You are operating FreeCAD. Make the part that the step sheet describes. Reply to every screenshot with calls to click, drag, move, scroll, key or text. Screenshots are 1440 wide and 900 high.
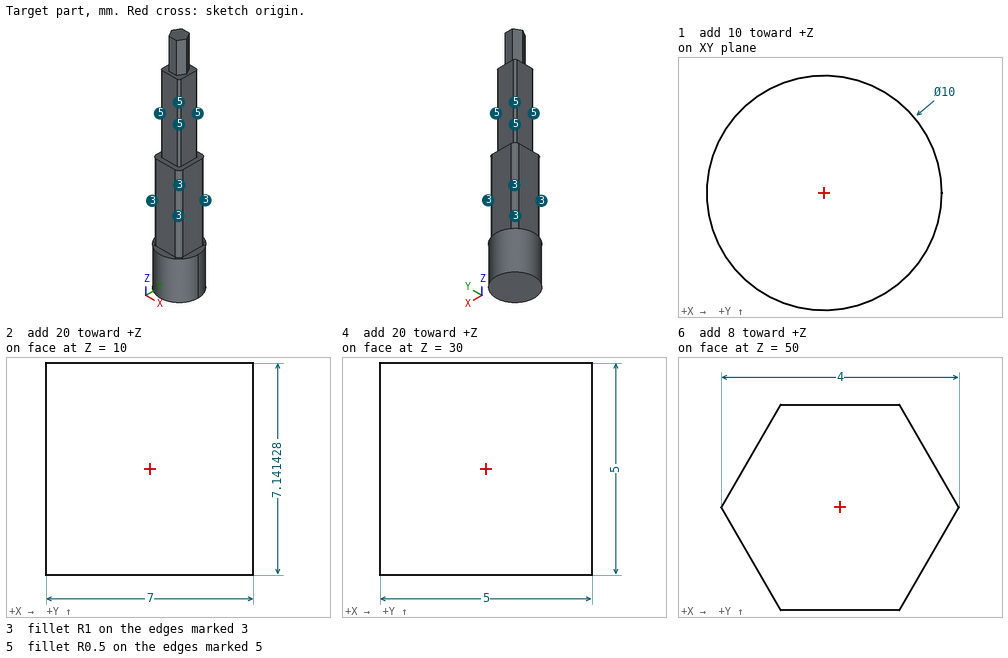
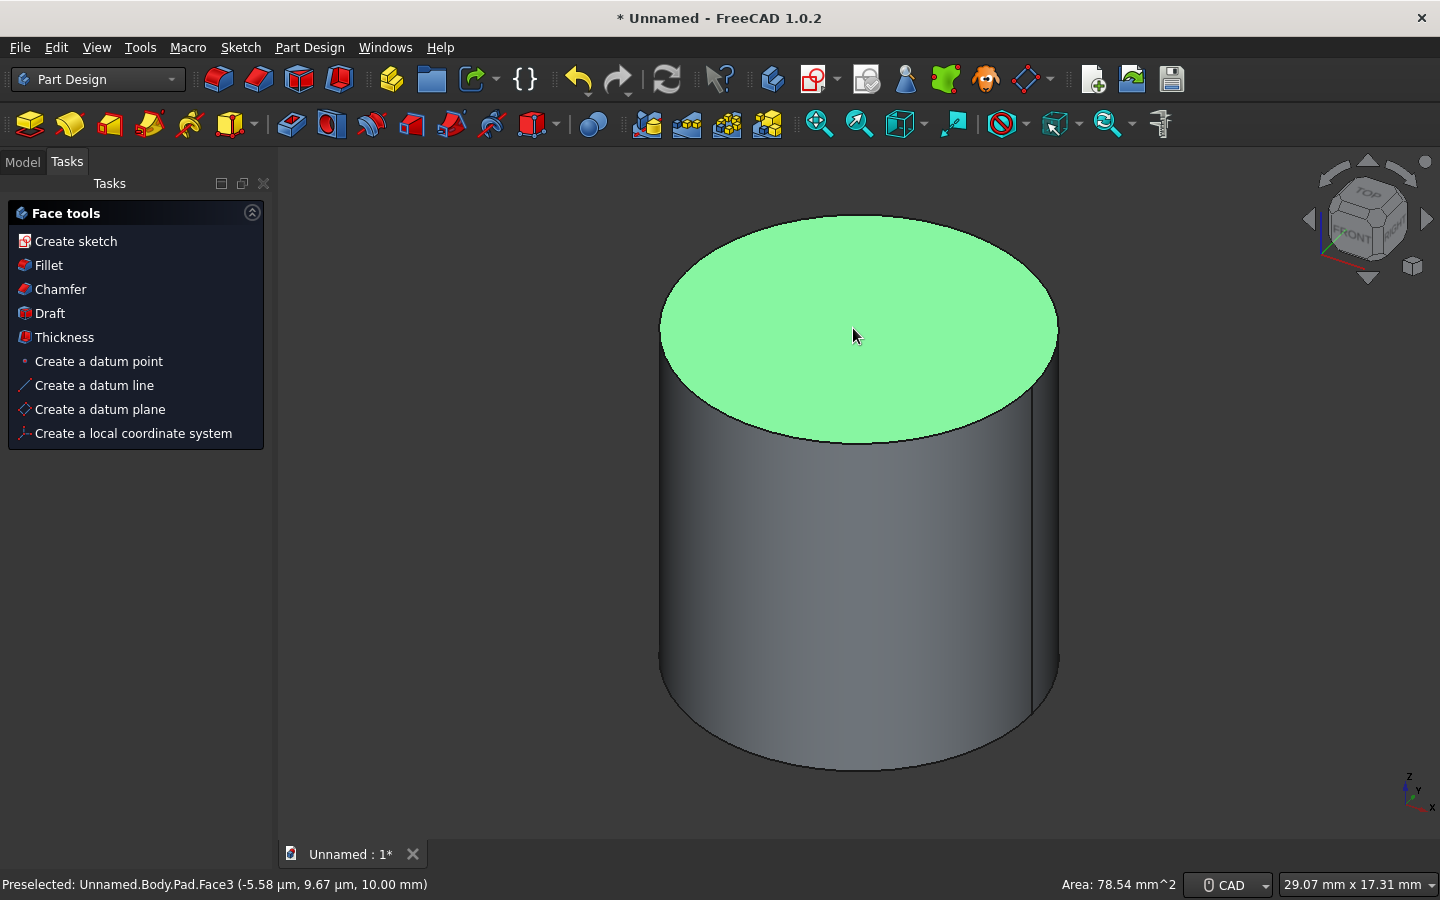
click(814, 80)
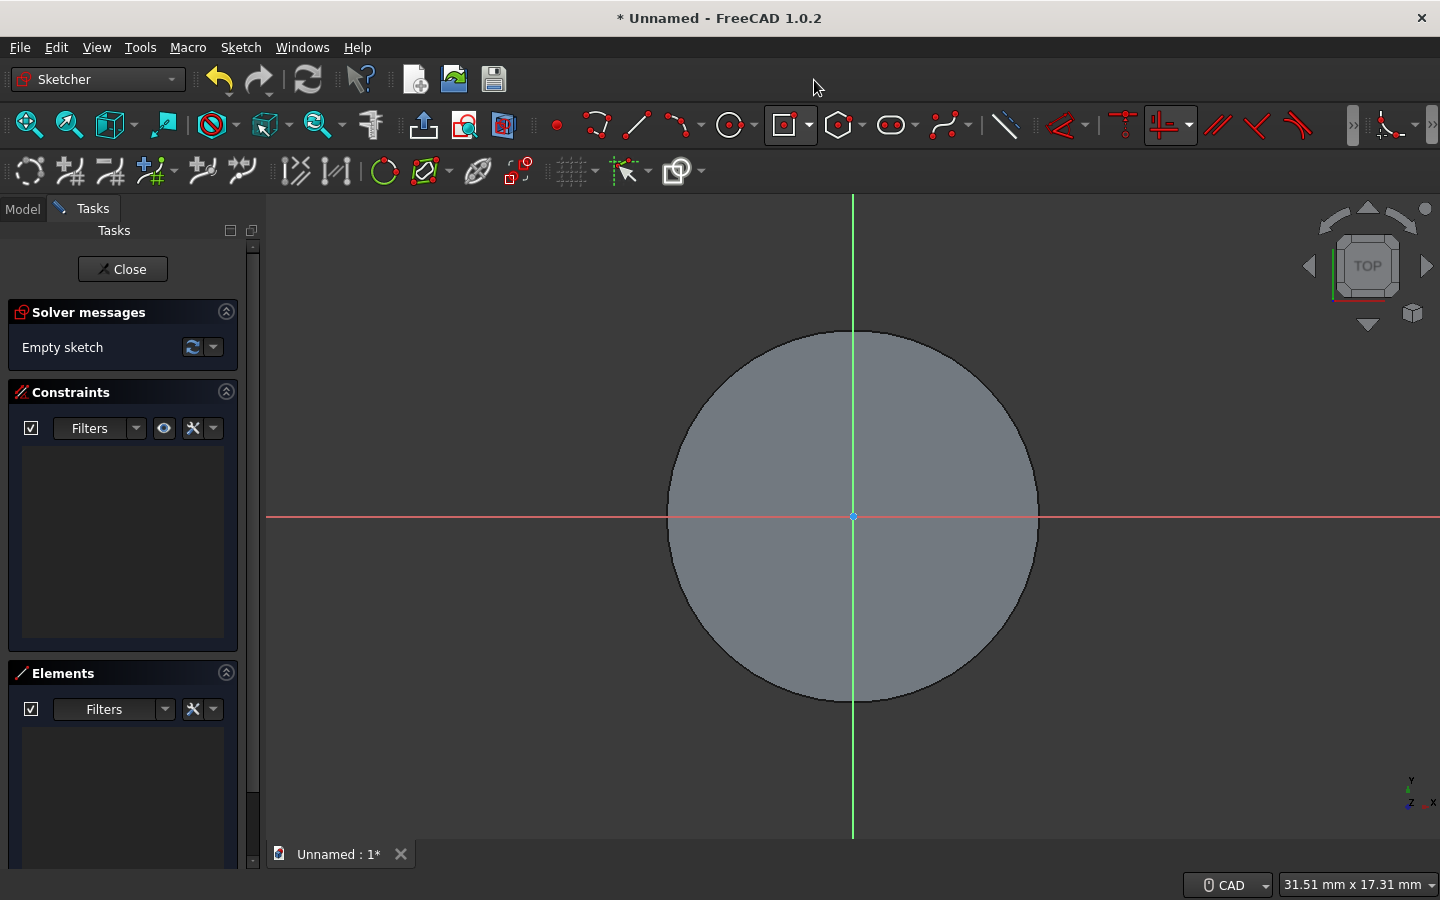
scroll(992, 517, up, 2)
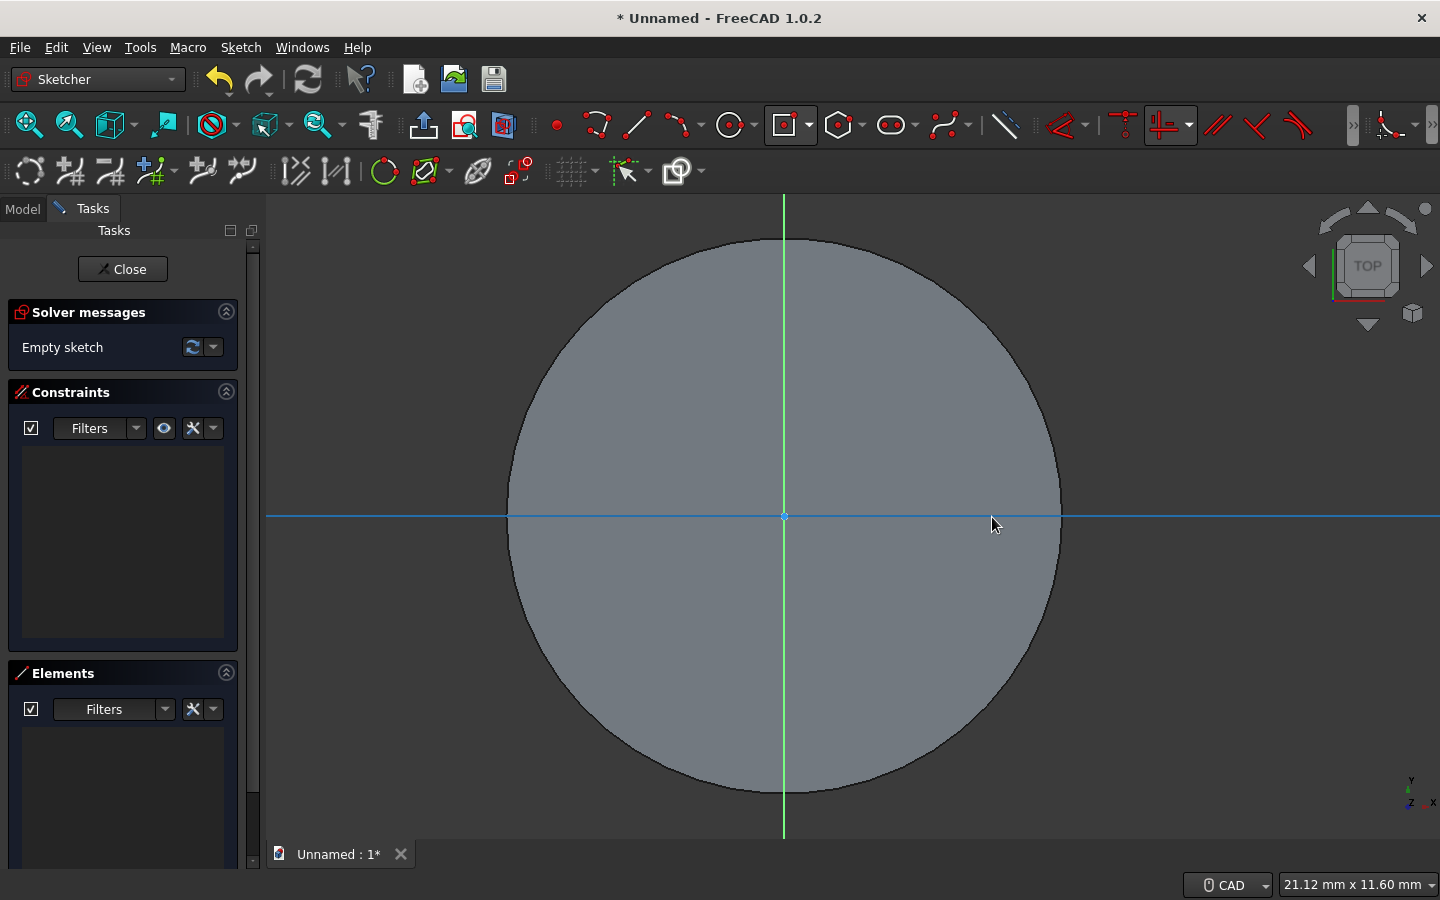
key(g)
key(v)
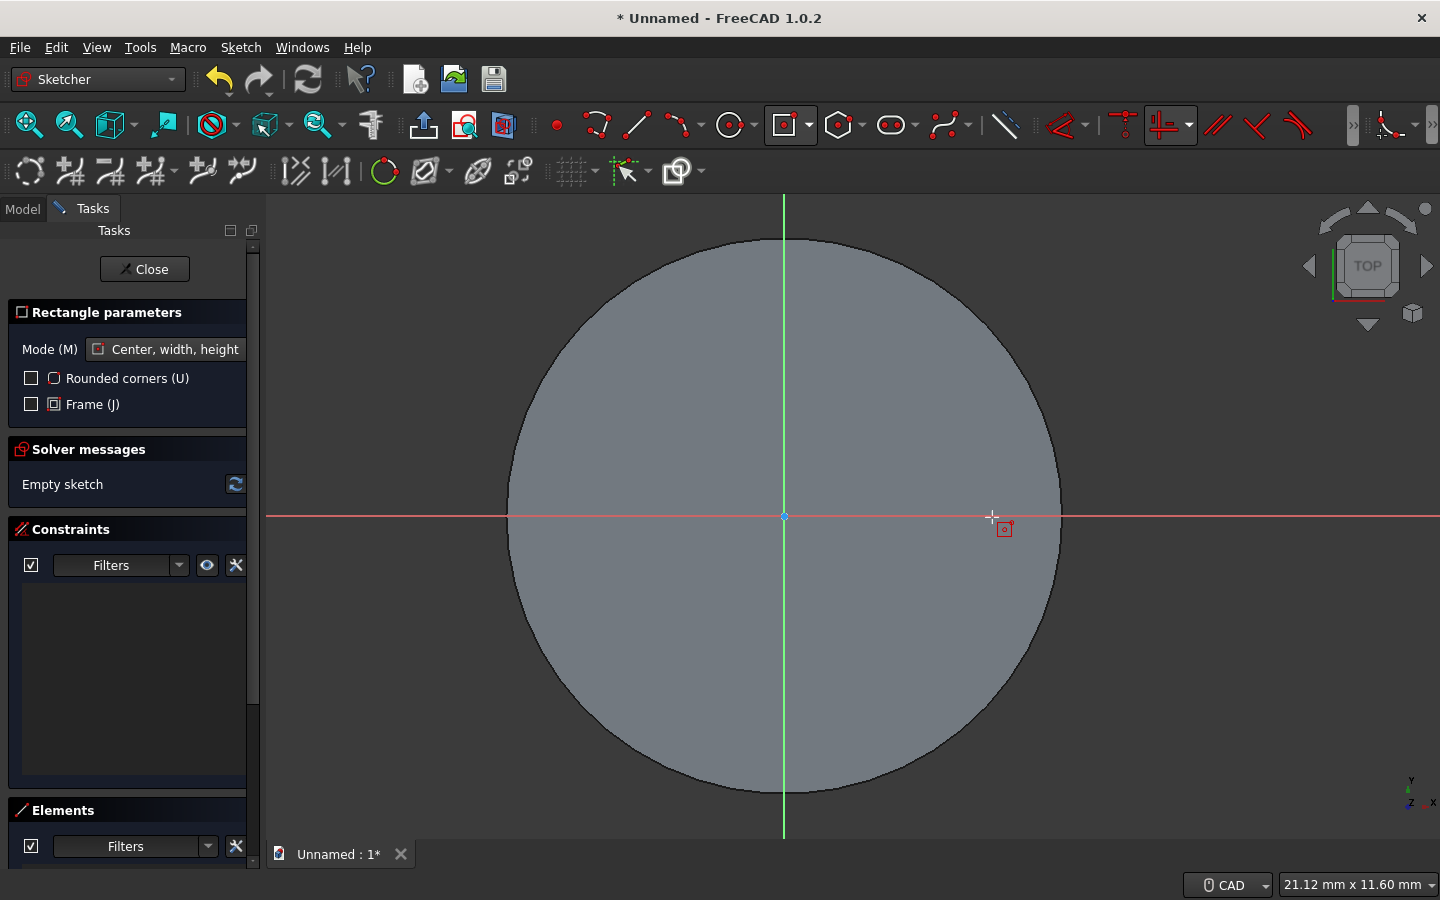
click(784, 516)
click(979, 318)
key(Escape)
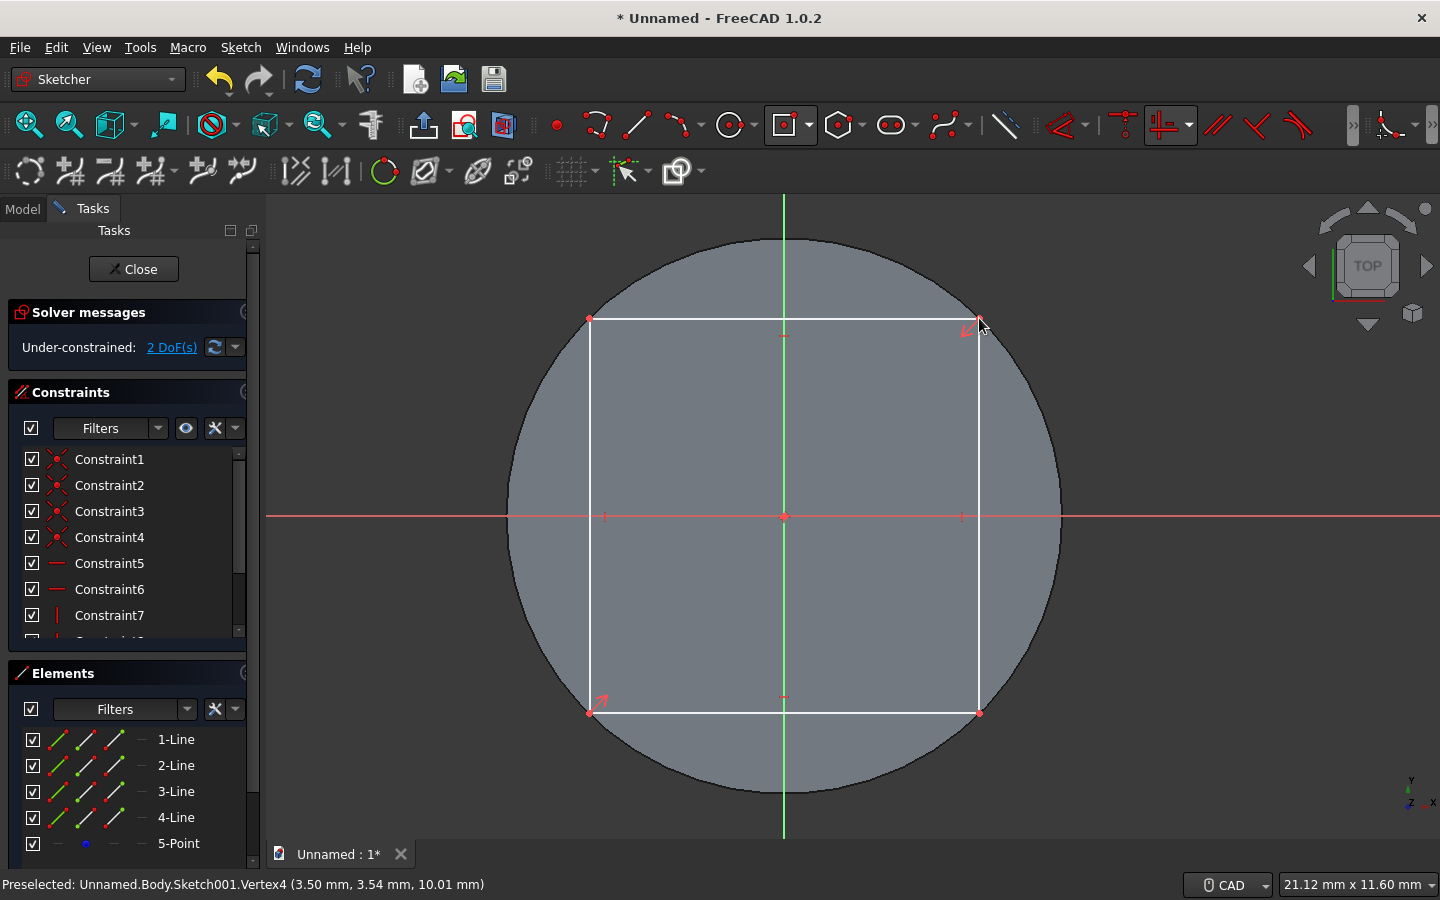
key(d)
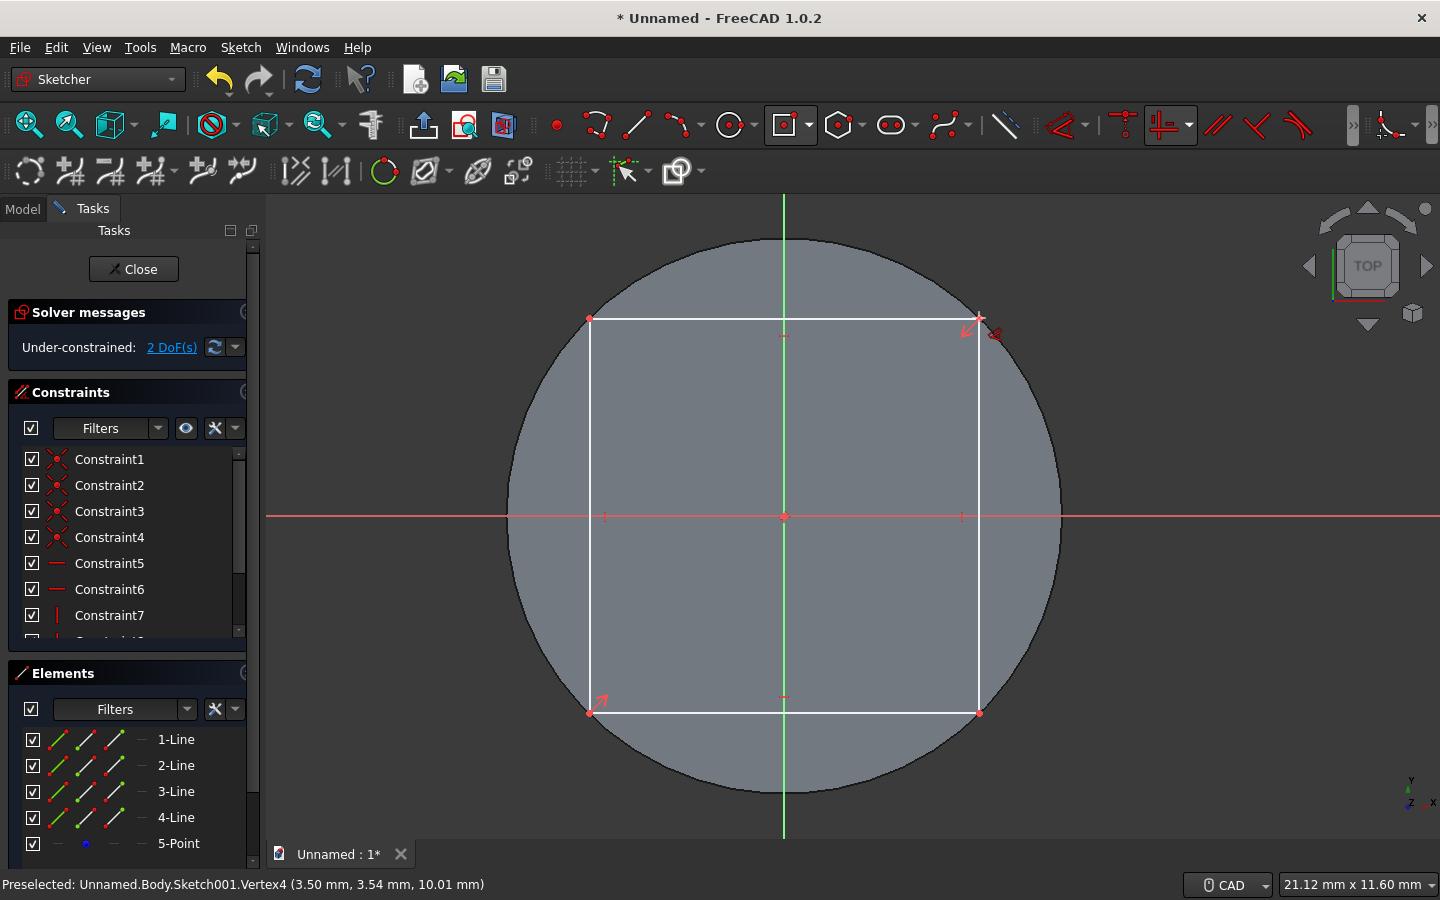
click(706, 713)
click(695, 747)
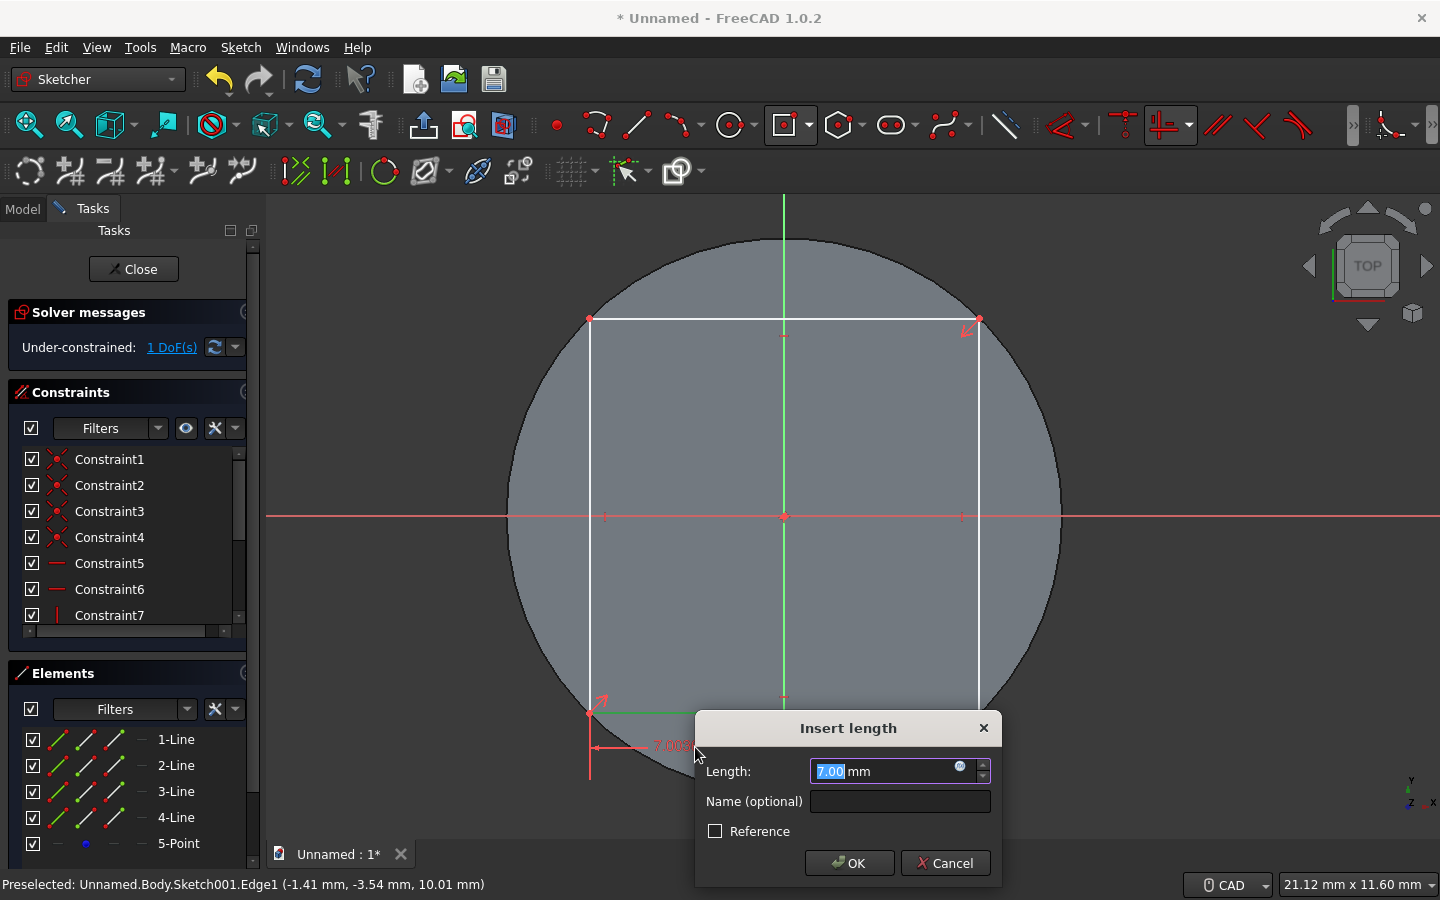
text(7)
key(Return)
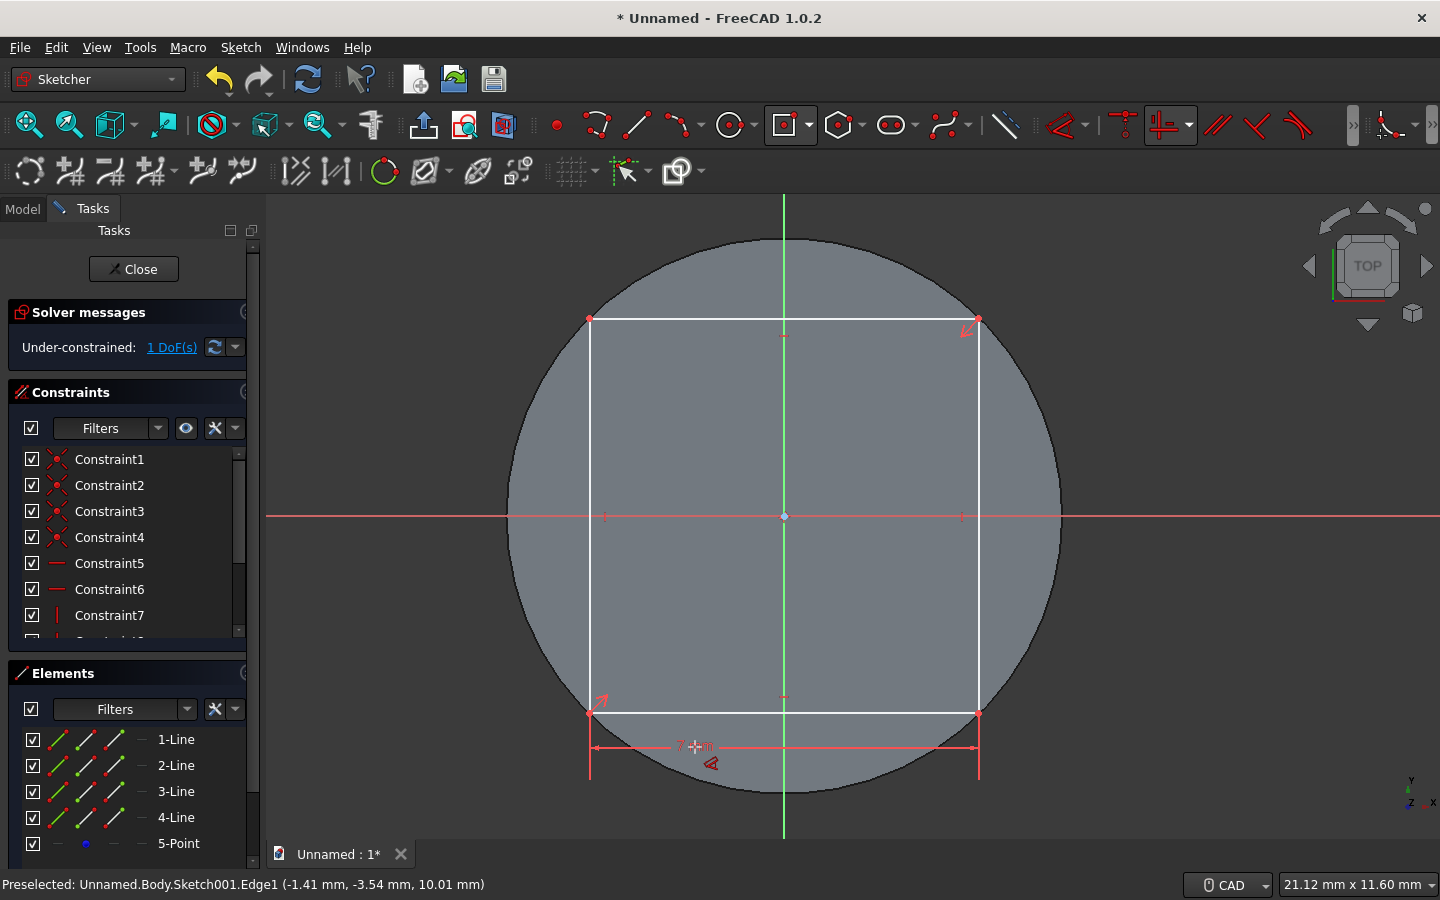
click(979, 595)
click(1013, 425)